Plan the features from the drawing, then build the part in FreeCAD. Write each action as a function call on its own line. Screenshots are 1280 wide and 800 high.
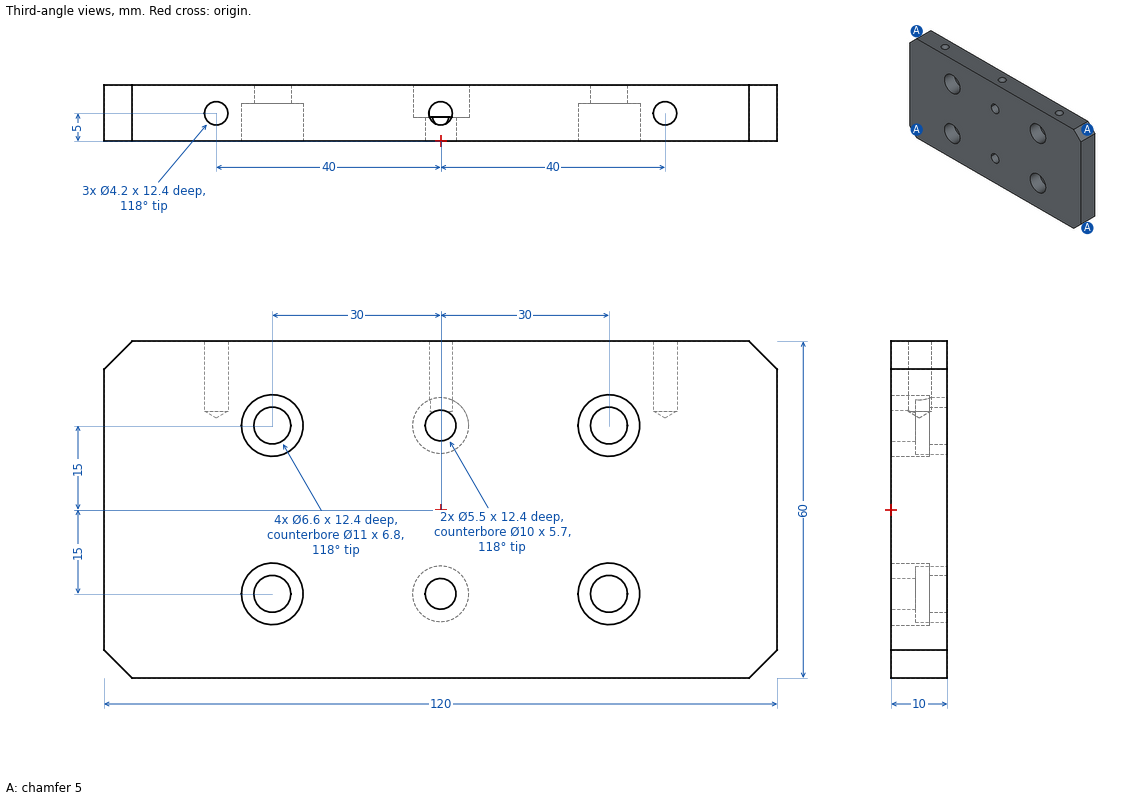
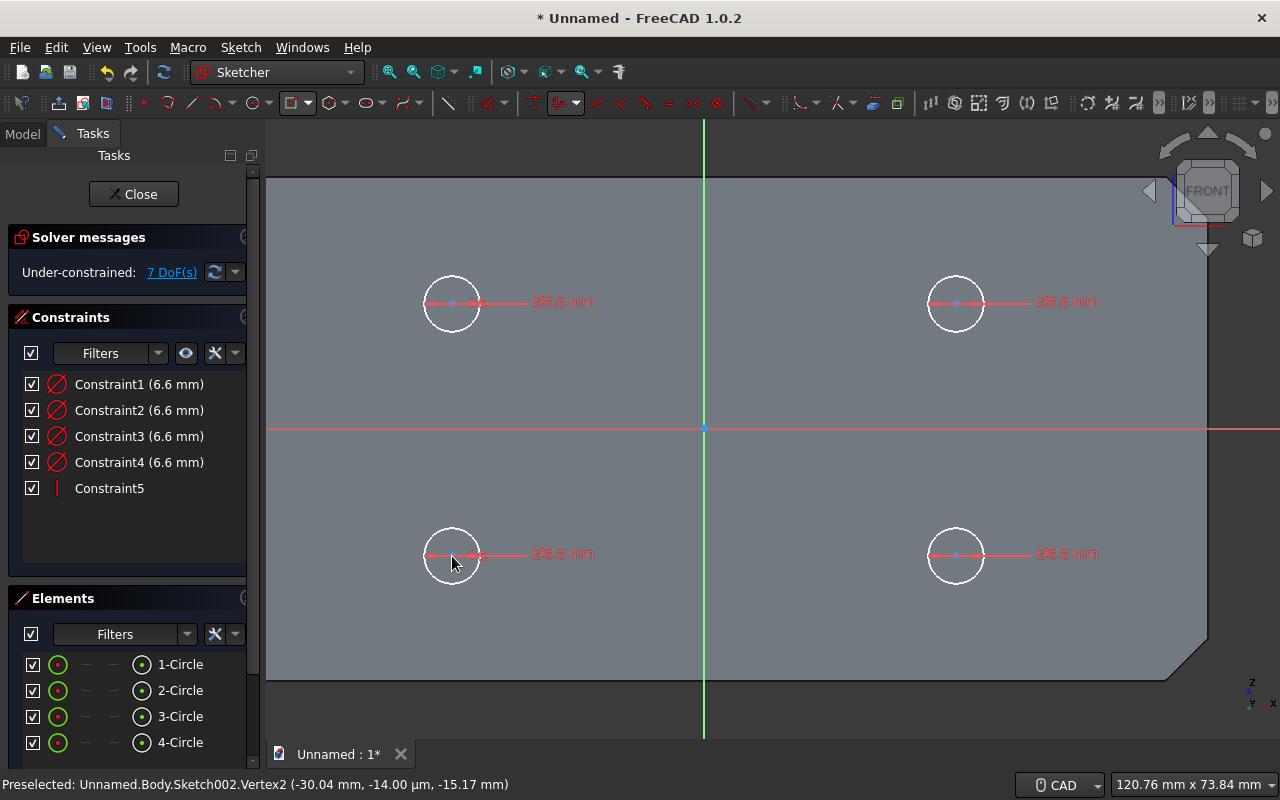
click(452, 304)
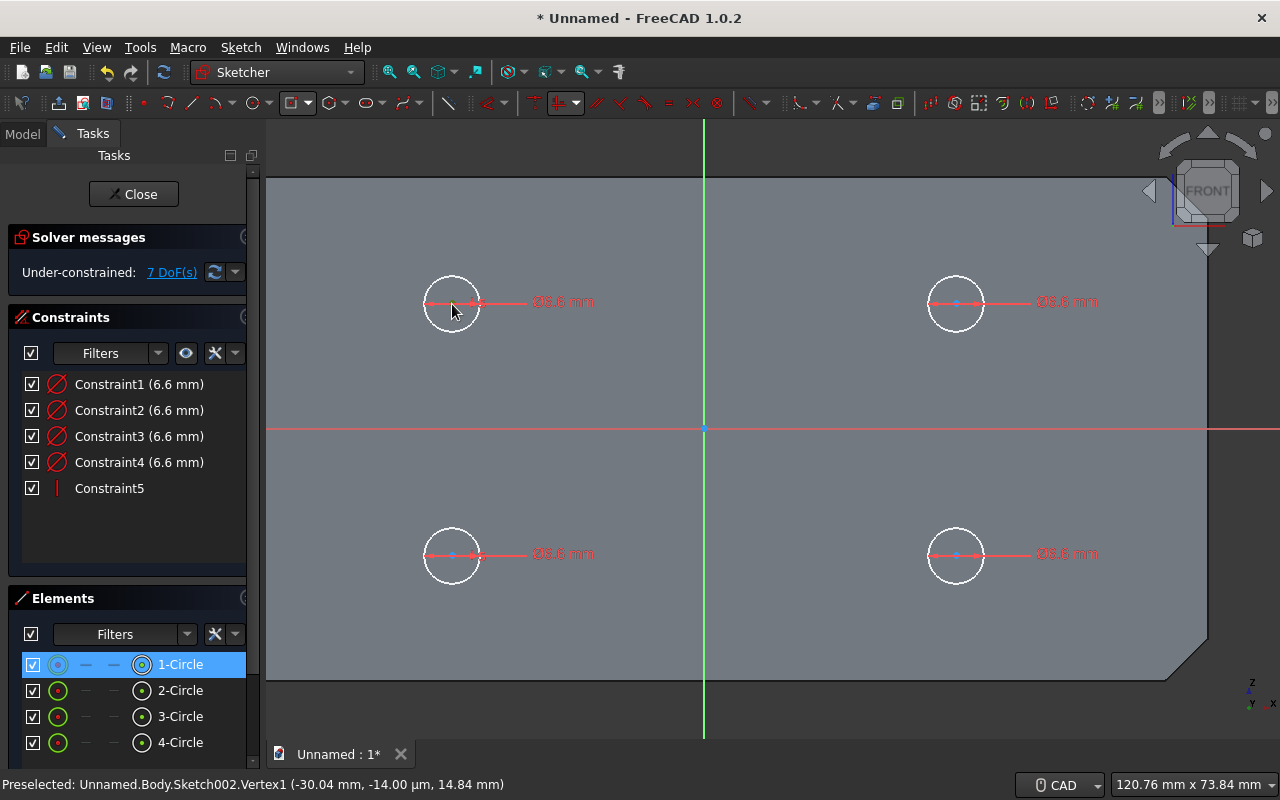
click(956, 304)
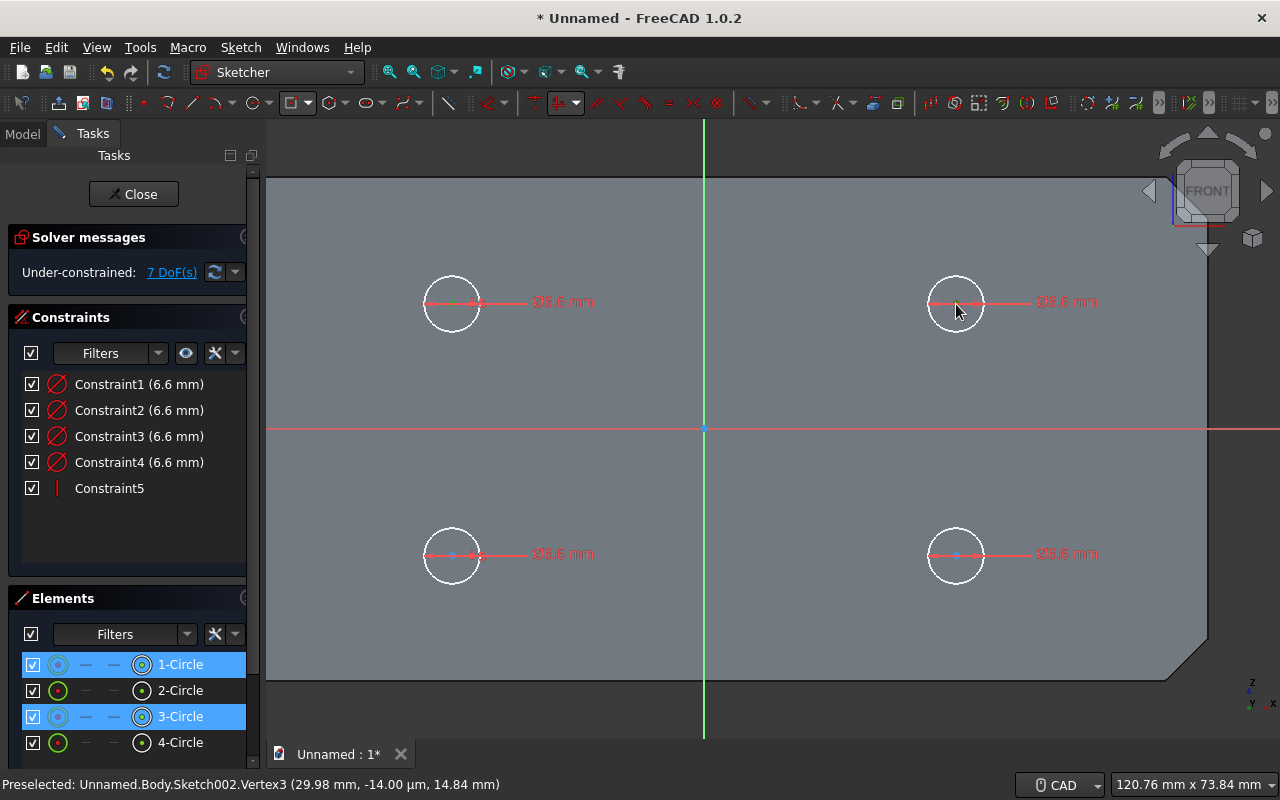
key(h)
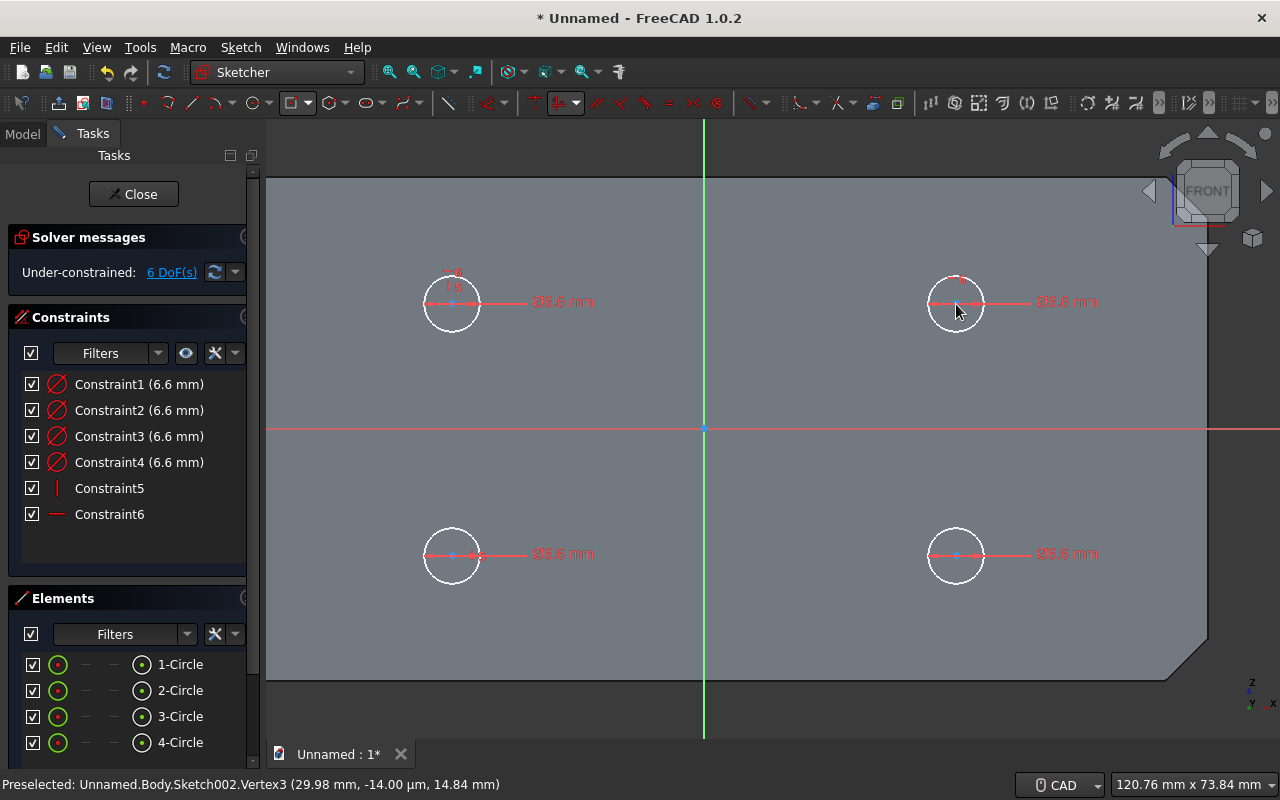
click(956, 304)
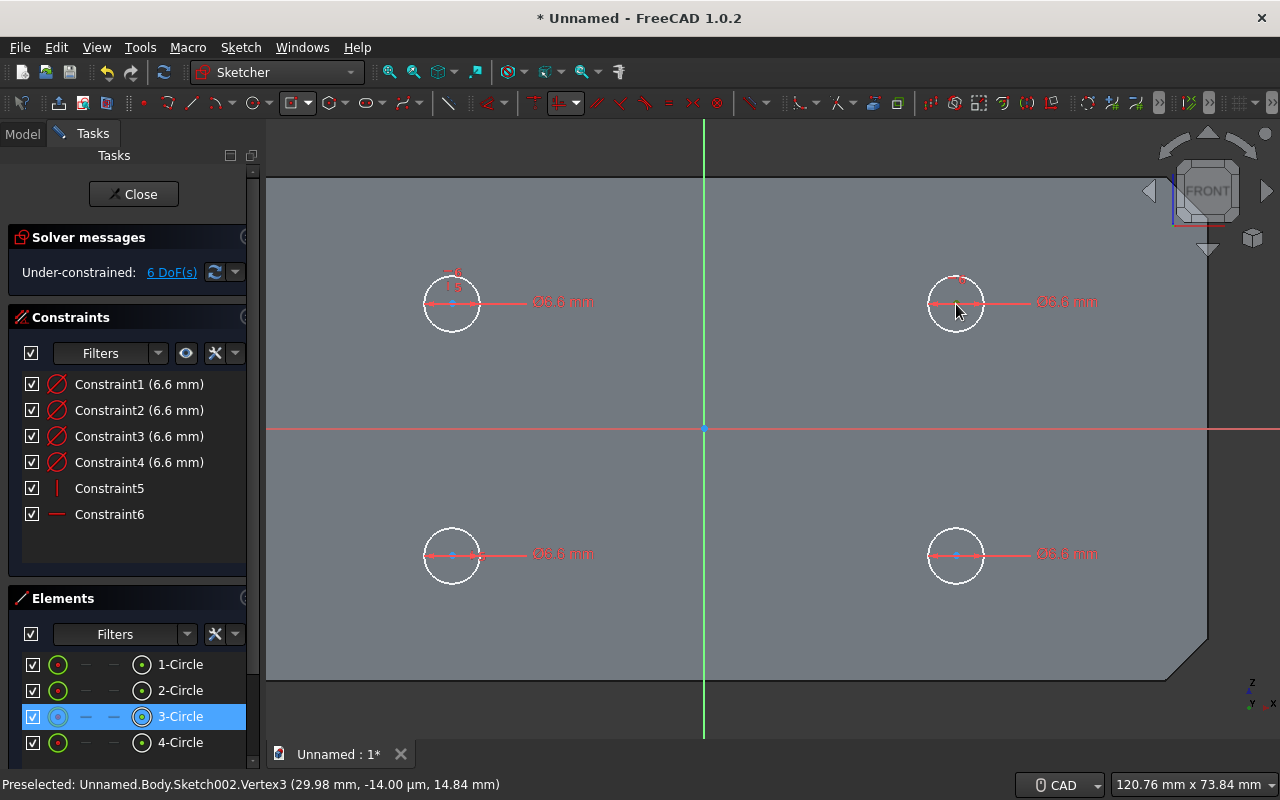
click(956, 556)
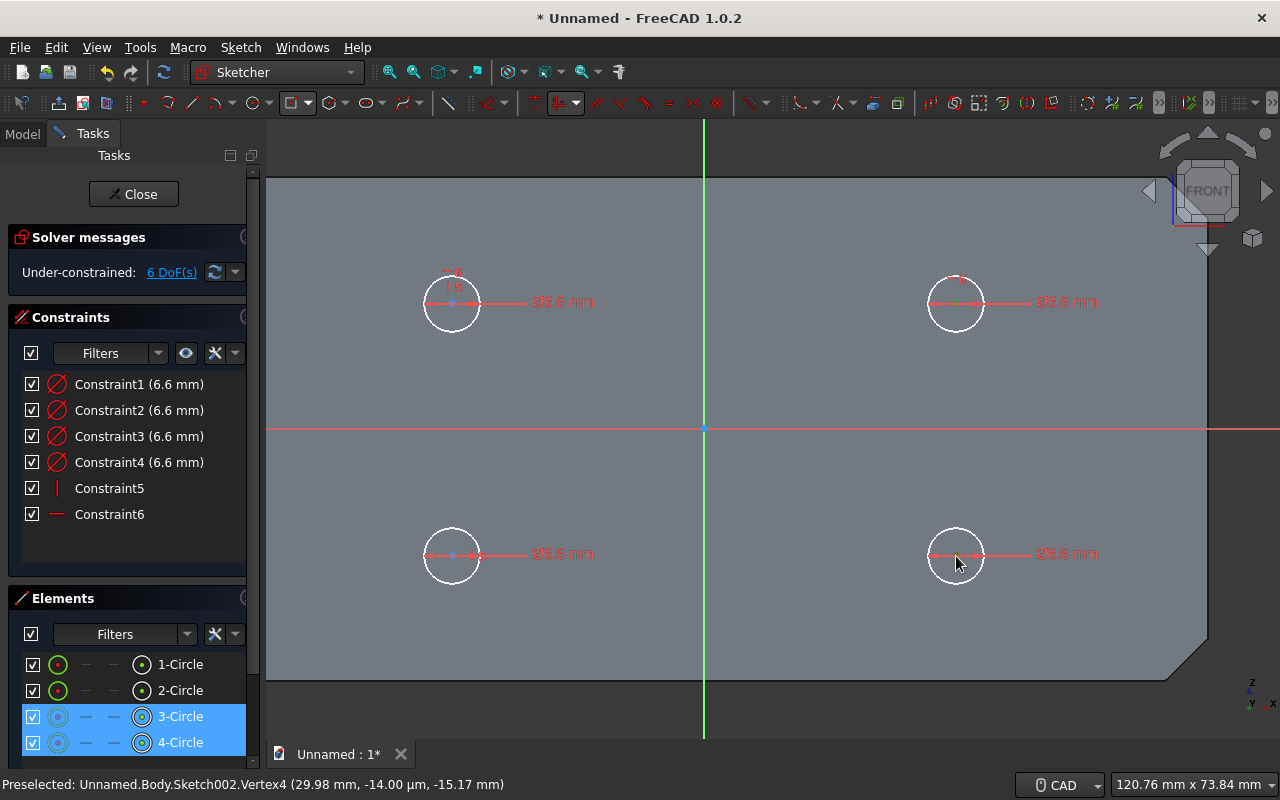
key(v)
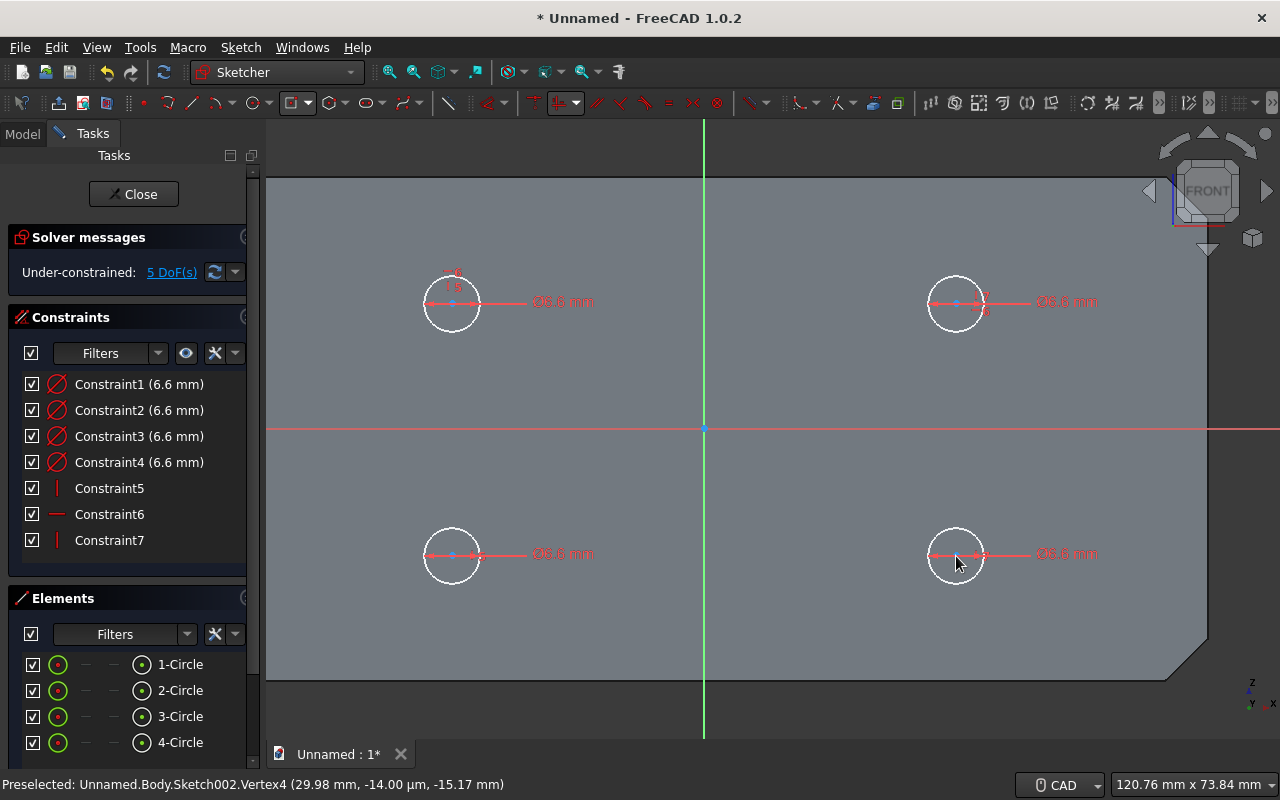
click(452, 556)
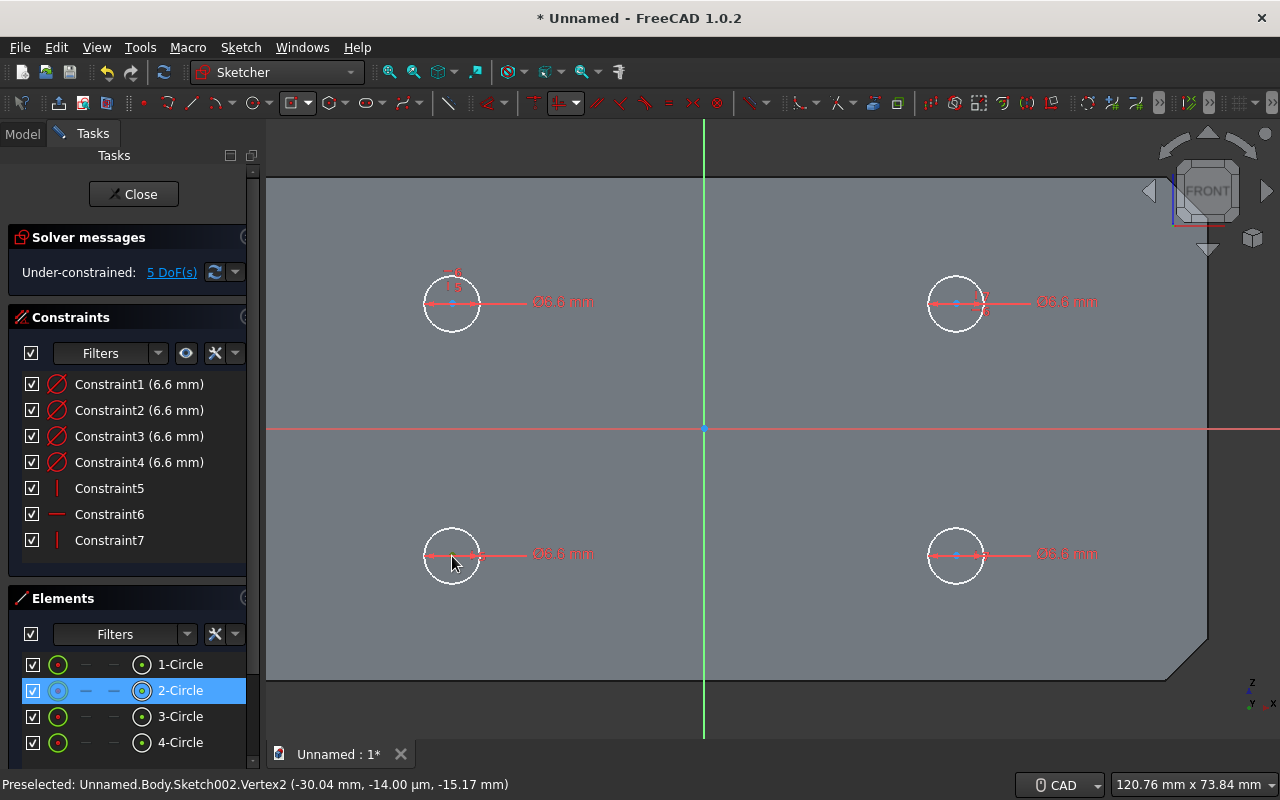
click(956, 556)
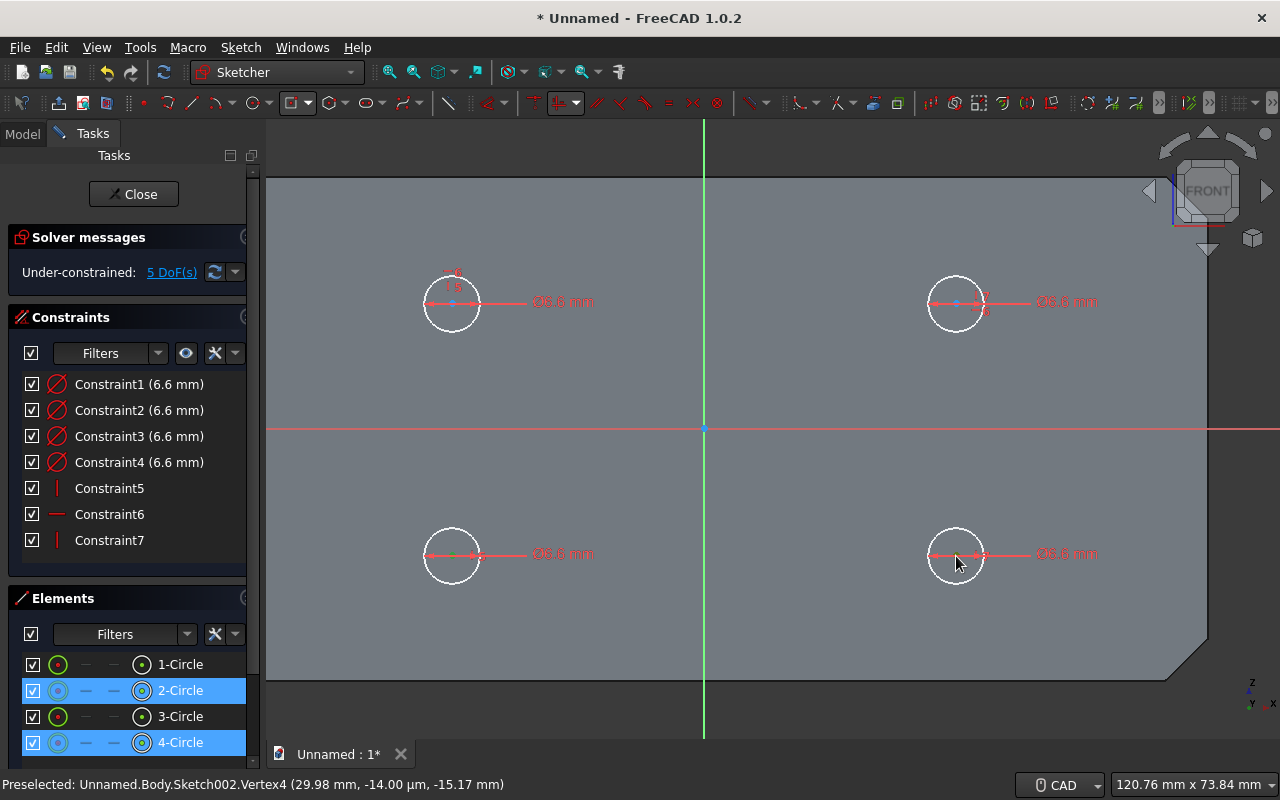
key(h)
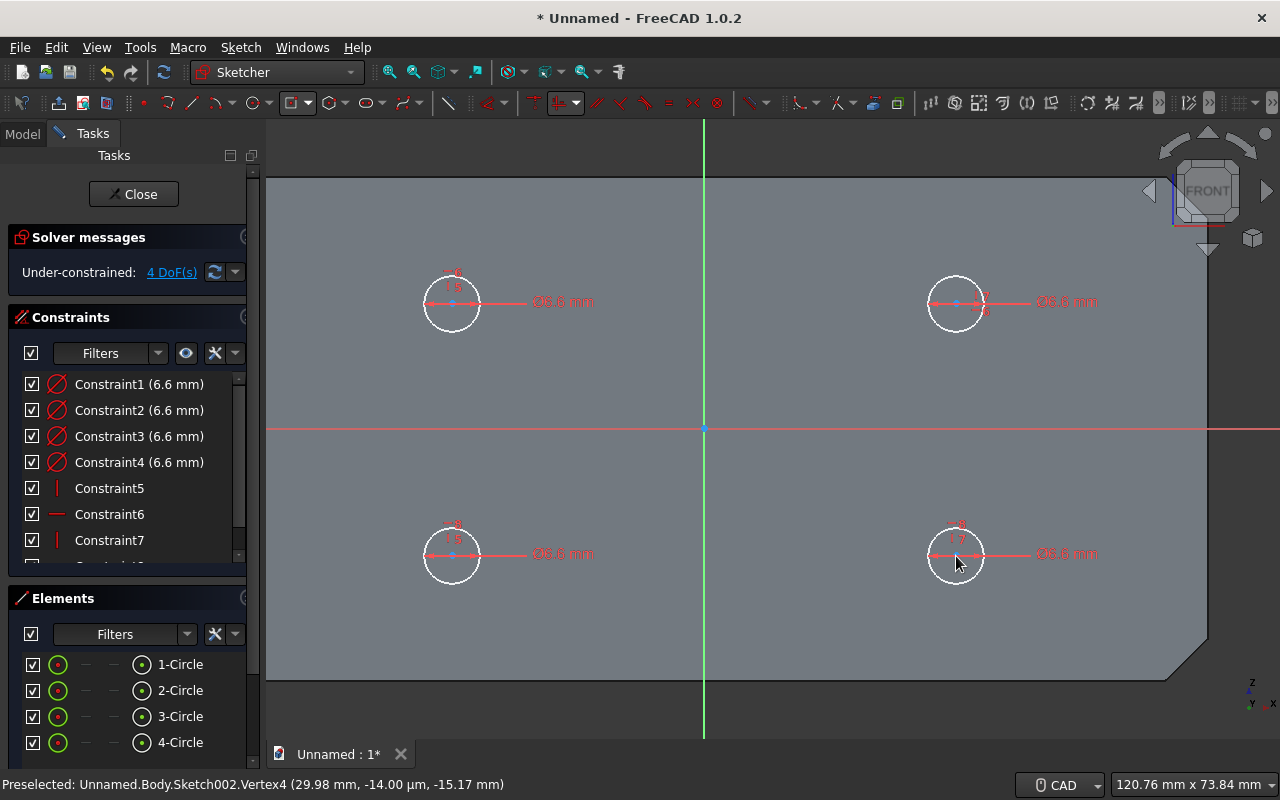
click(452, 304)